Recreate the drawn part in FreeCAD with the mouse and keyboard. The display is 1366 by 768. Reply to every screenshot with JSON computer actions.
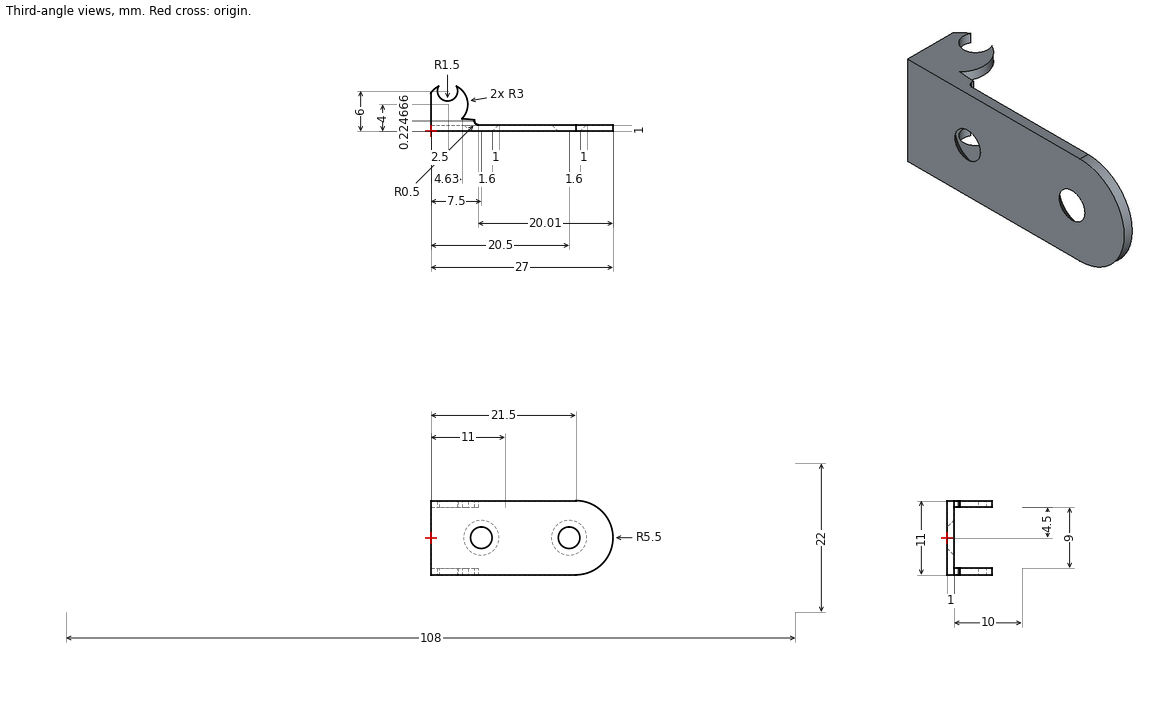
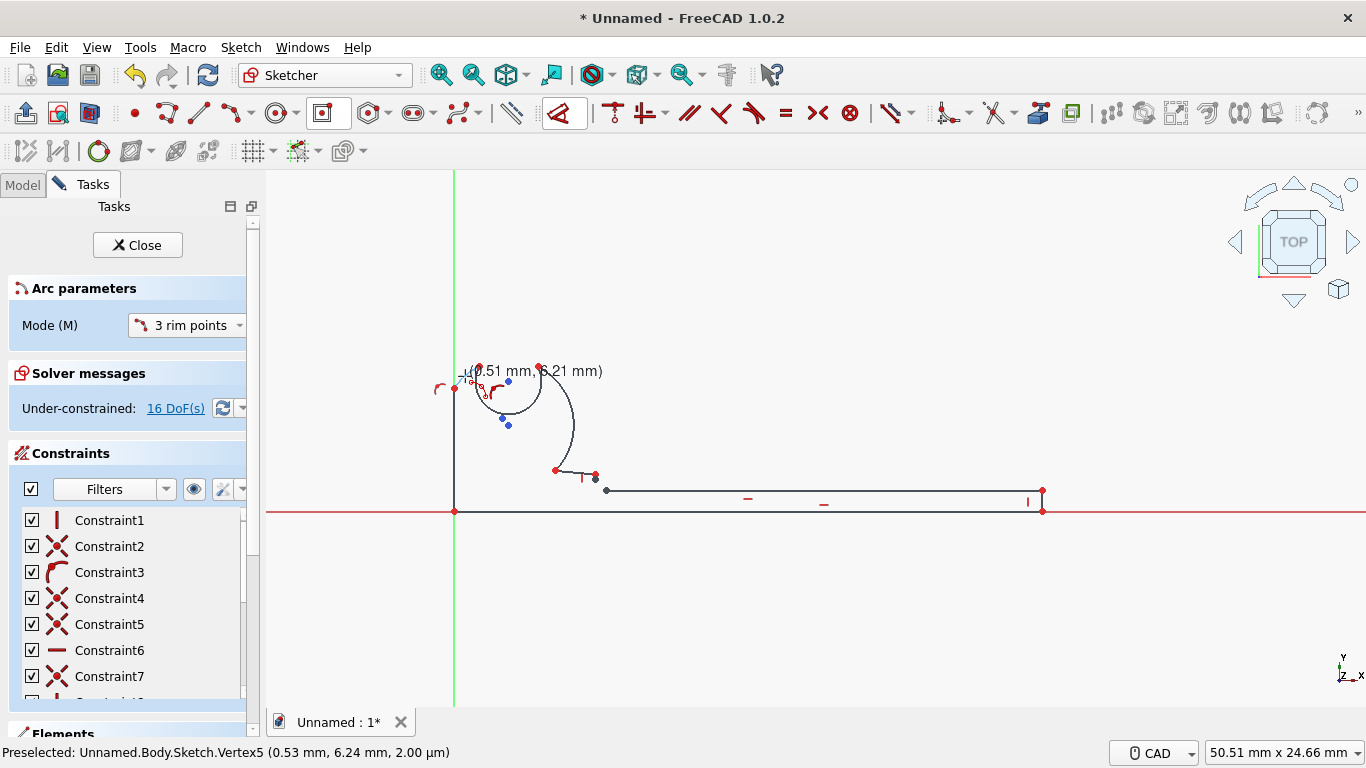
{"action": "left_click", "coordinate": [606, 491]}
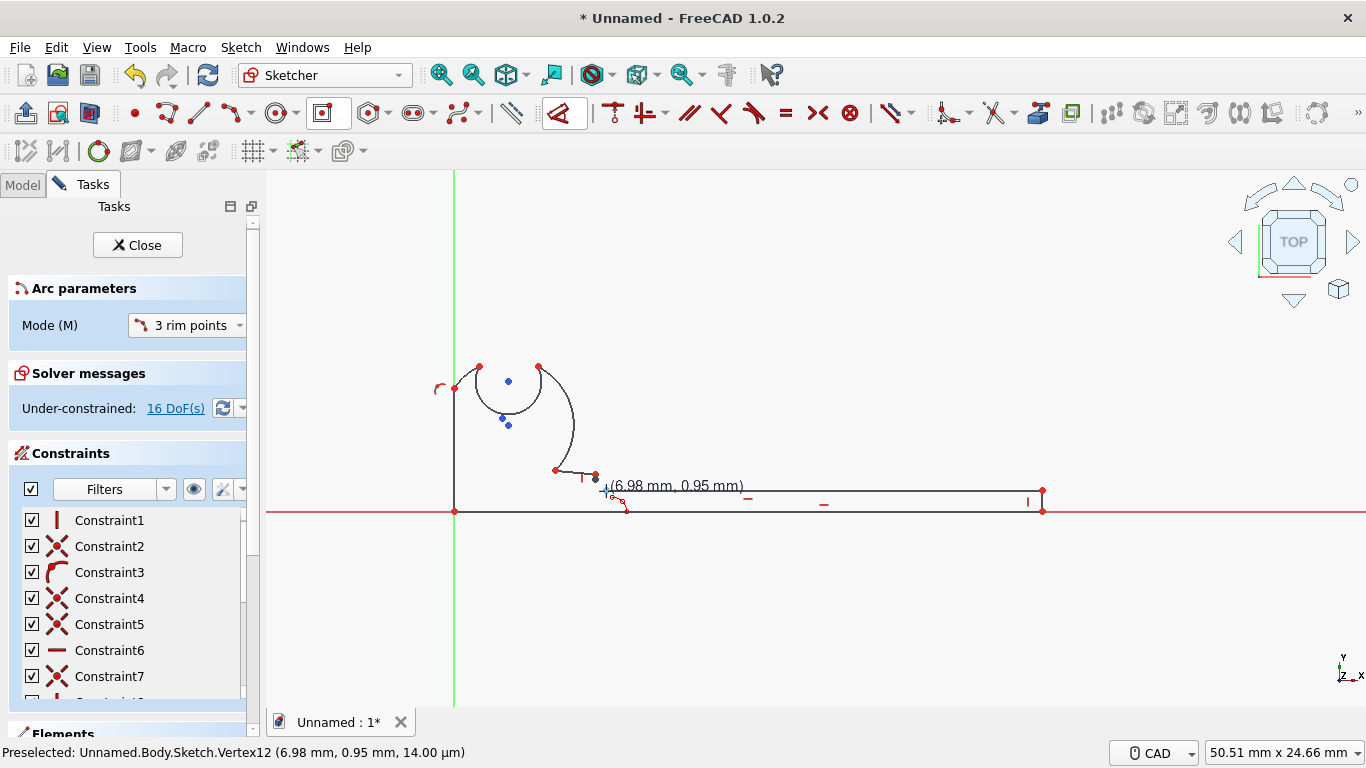
{"action": "scroll", "coordinate": [595, 479], "scroll_direction": "up", "scroll_amount": 10}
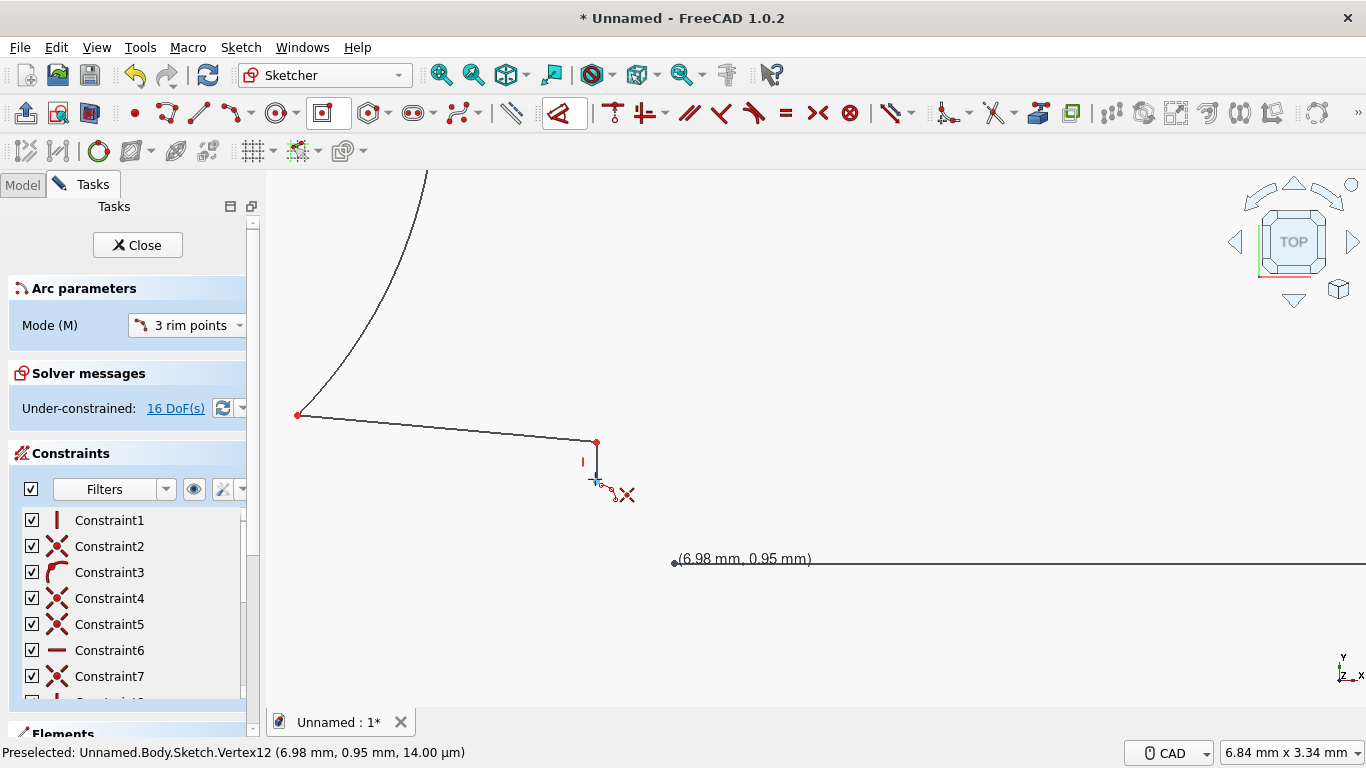
{"action": "left_click", "coordinate": [597, 481]}
{"action": "left_click", "coordinate": [620, 532]}
{"action": "key", "text": "Escape"}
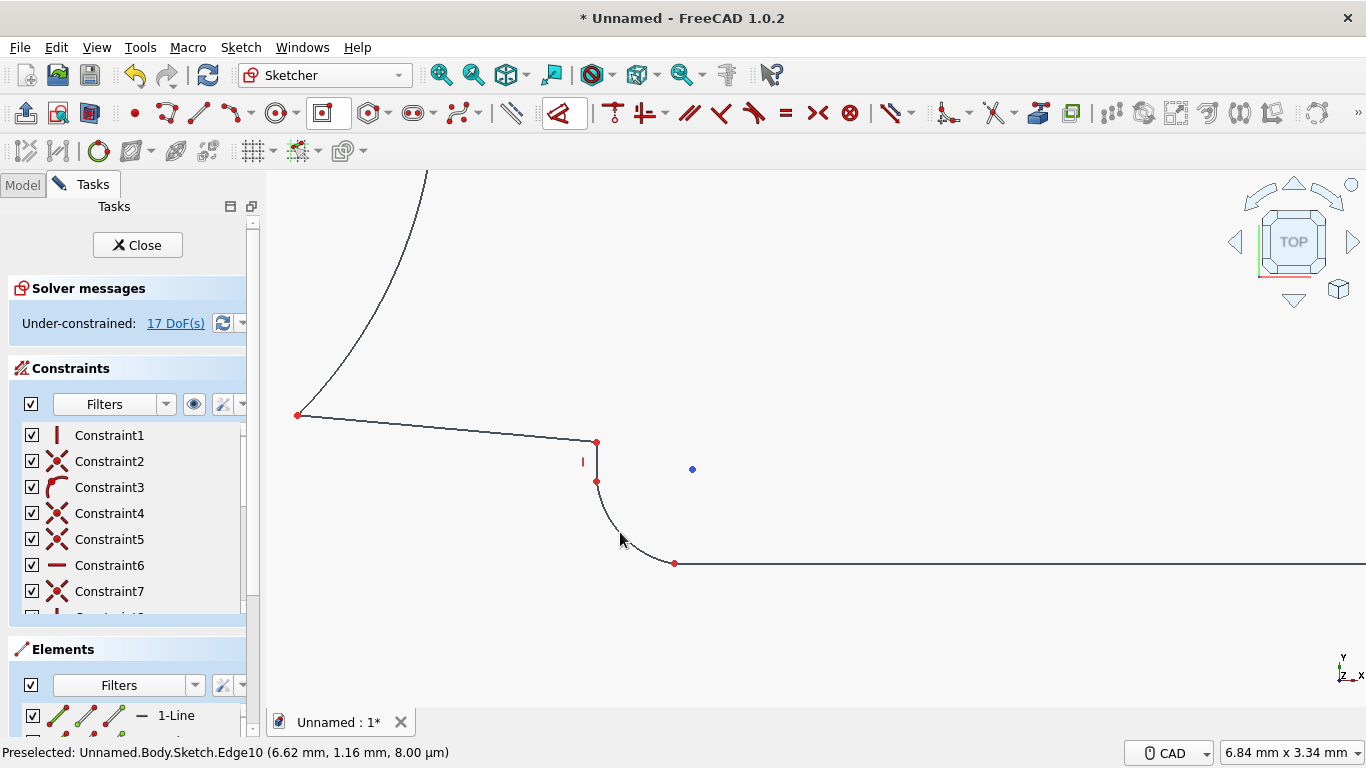
{"action": "left_click", "coordinate": [597, 469]}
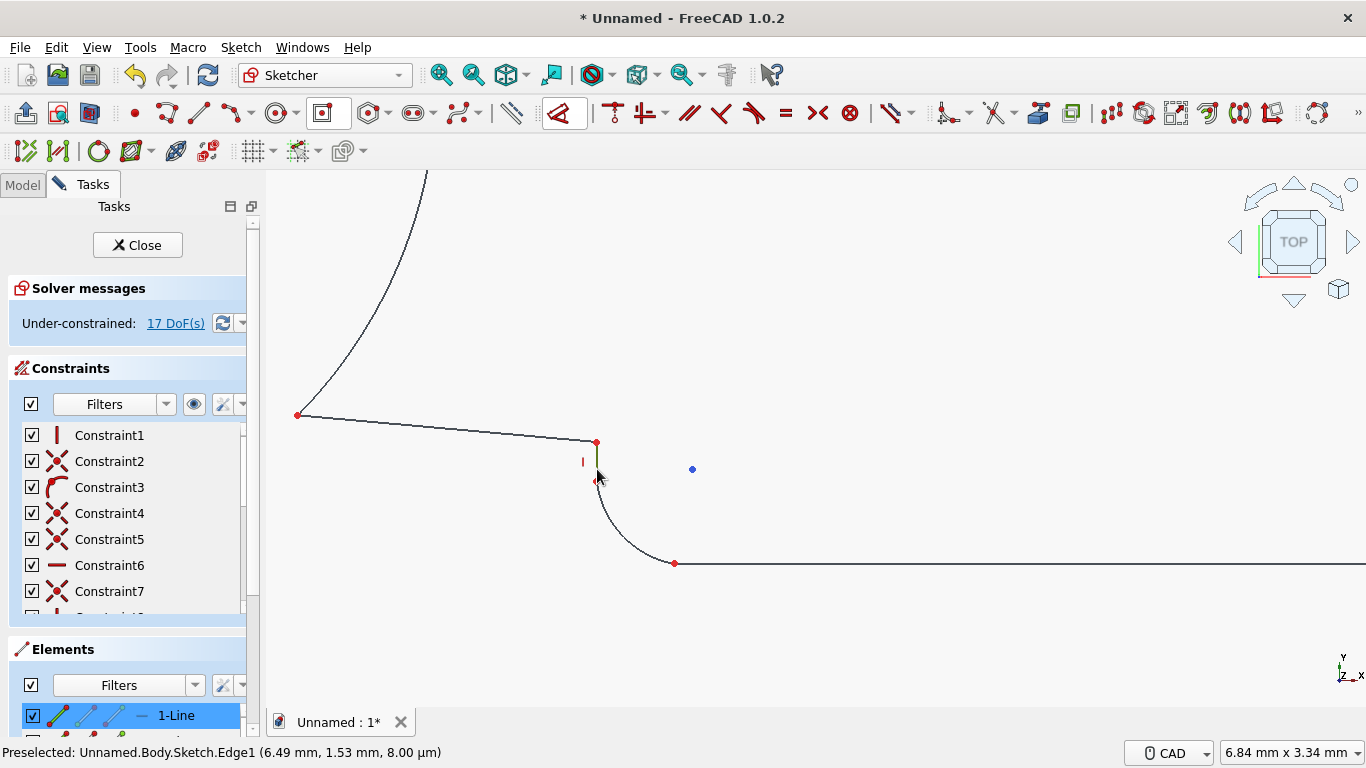
{"action": "left_click", "coordinate": [608, 516]}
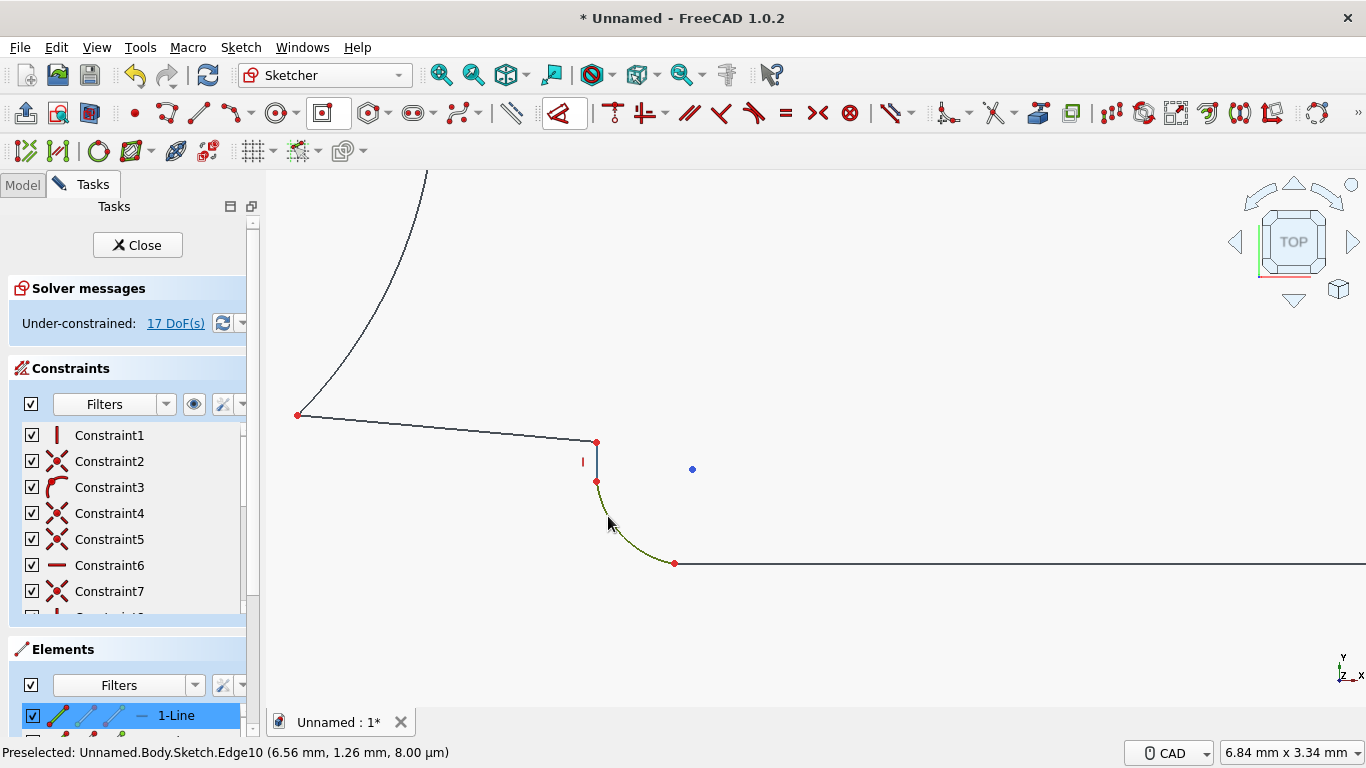
{"action": "key", "text": "t"}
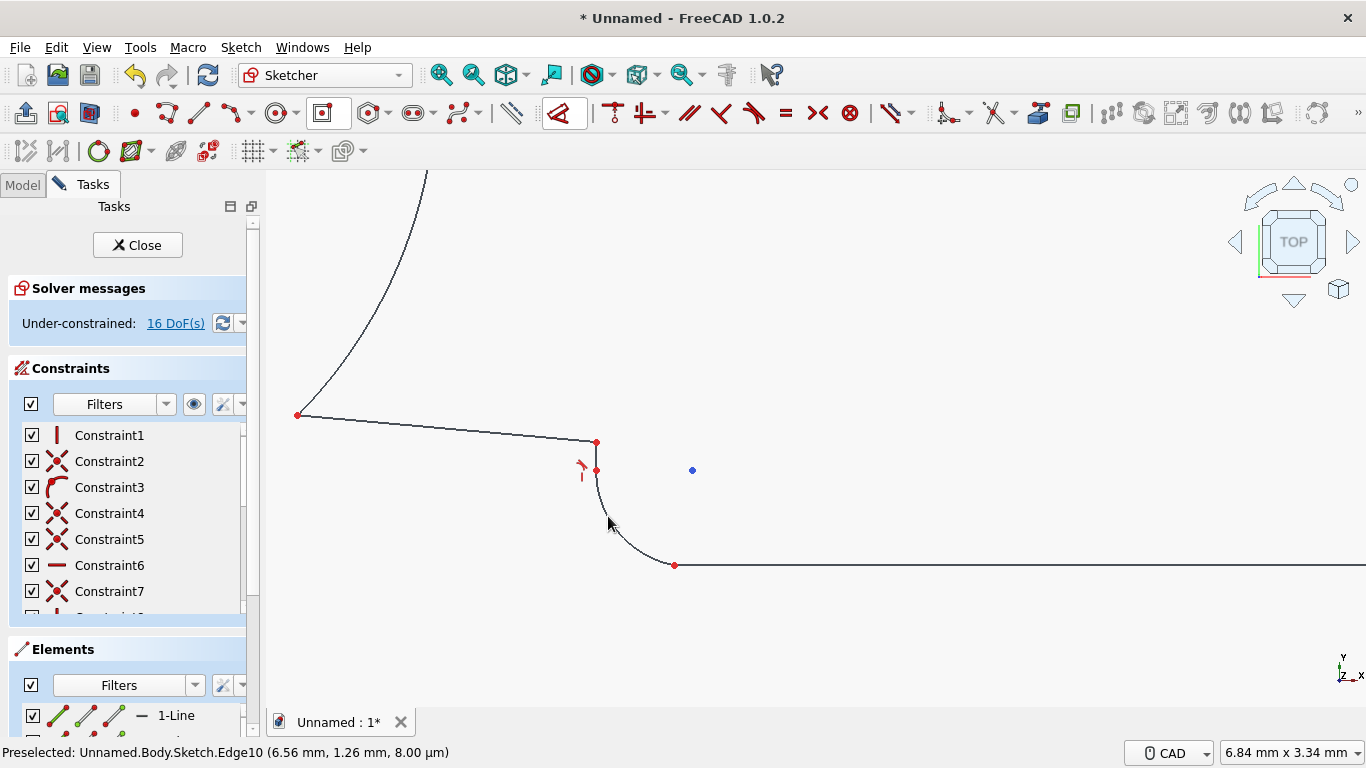
{"action": "scroll", "coordinate": [595, 479], "scroll_direction": "down", "scroll_amount": 10}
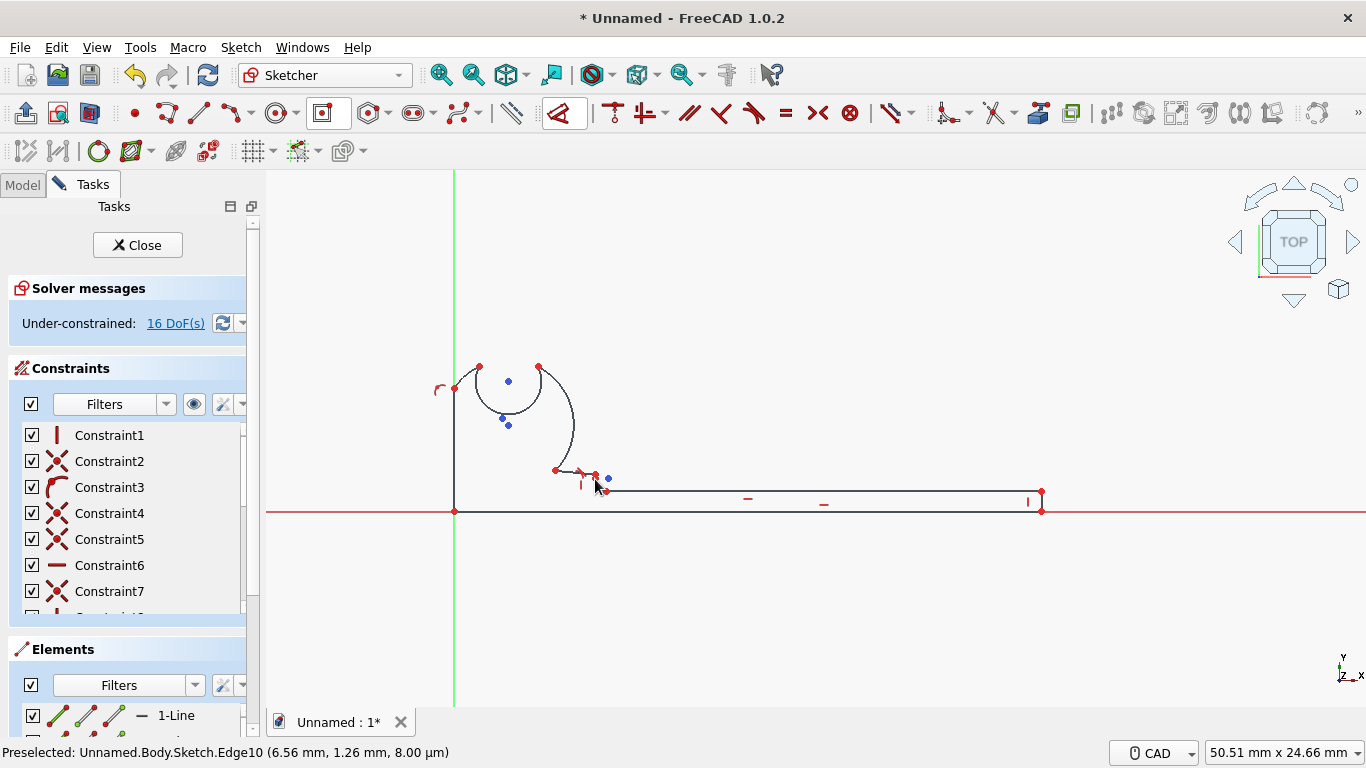
{"action": "left_click", "coordinate": [911, 491]}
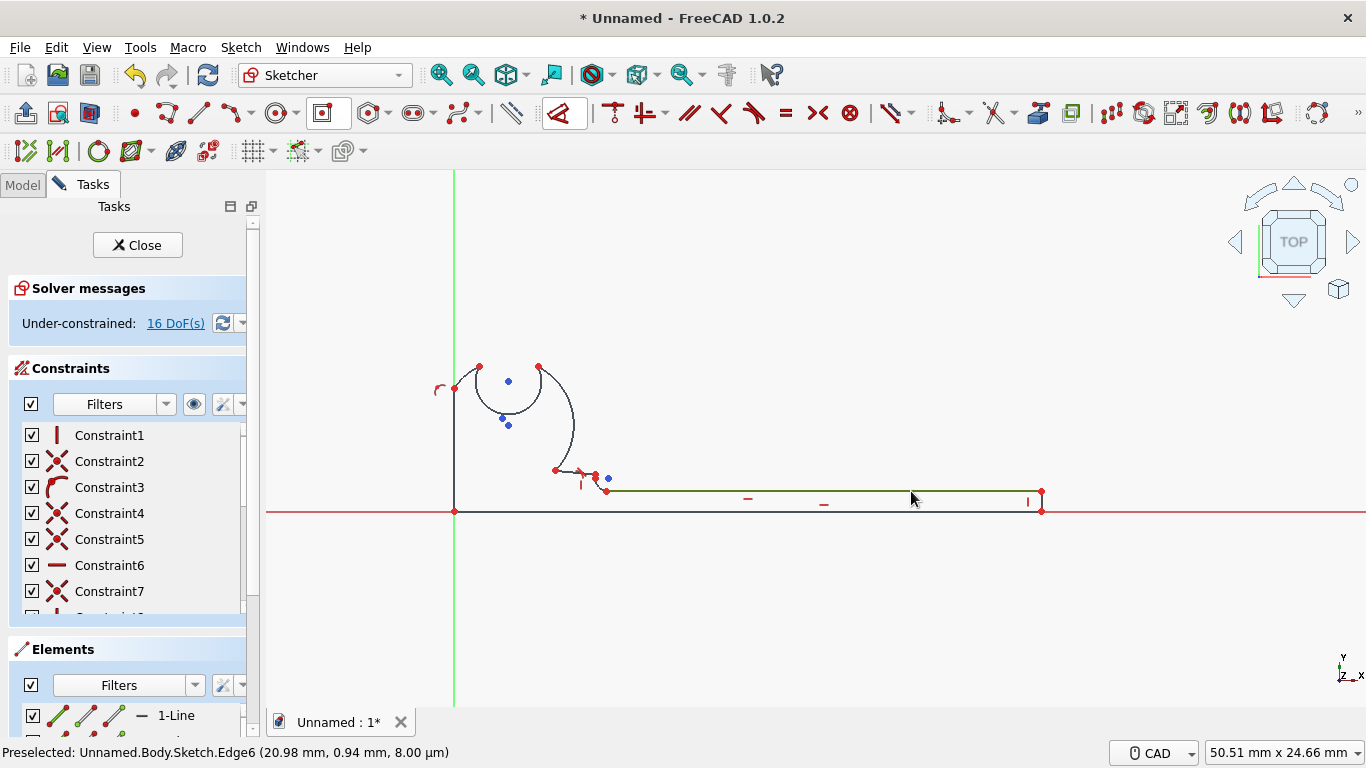
{"action": "scroll", "coordinate": [598, 487], "scroll_direction": "up", "scroll_amount": 3}